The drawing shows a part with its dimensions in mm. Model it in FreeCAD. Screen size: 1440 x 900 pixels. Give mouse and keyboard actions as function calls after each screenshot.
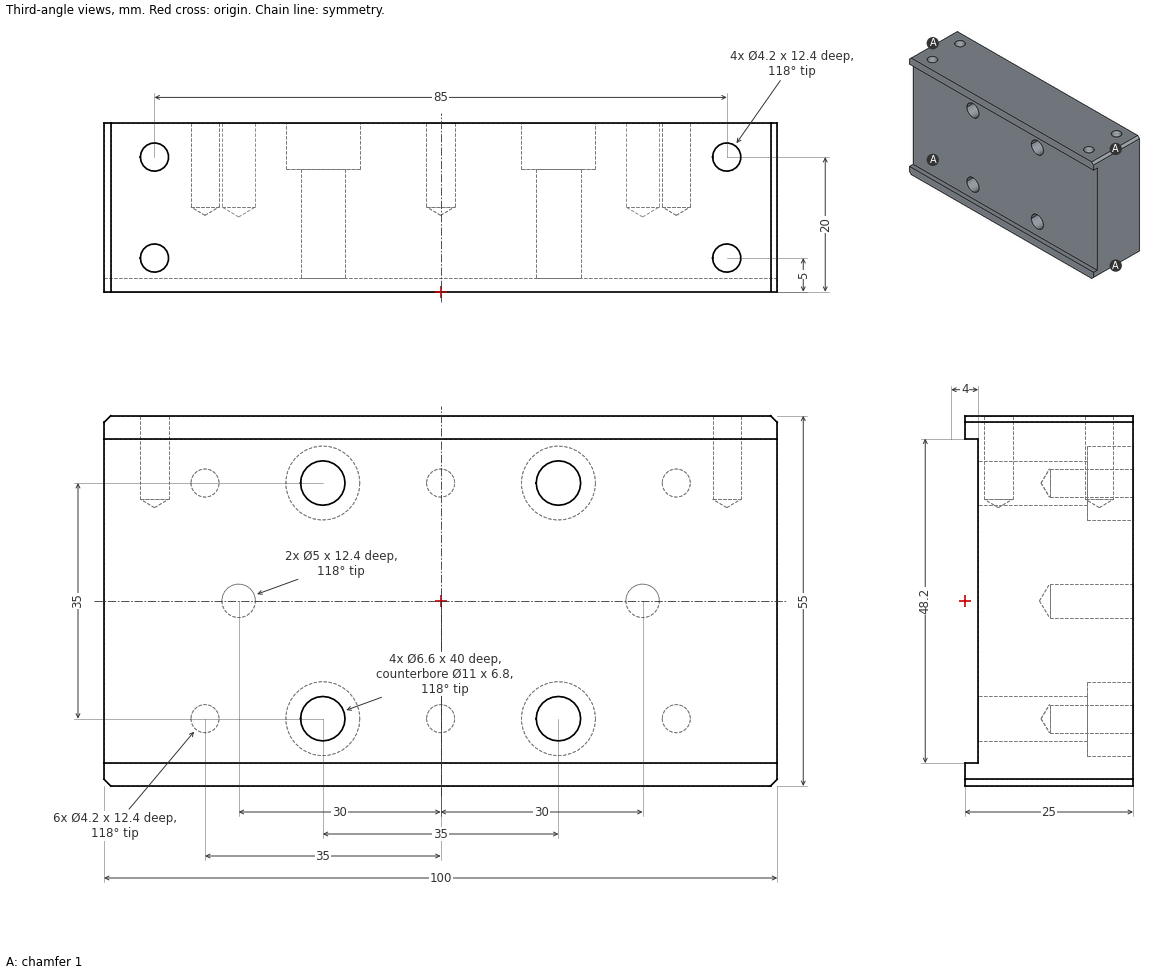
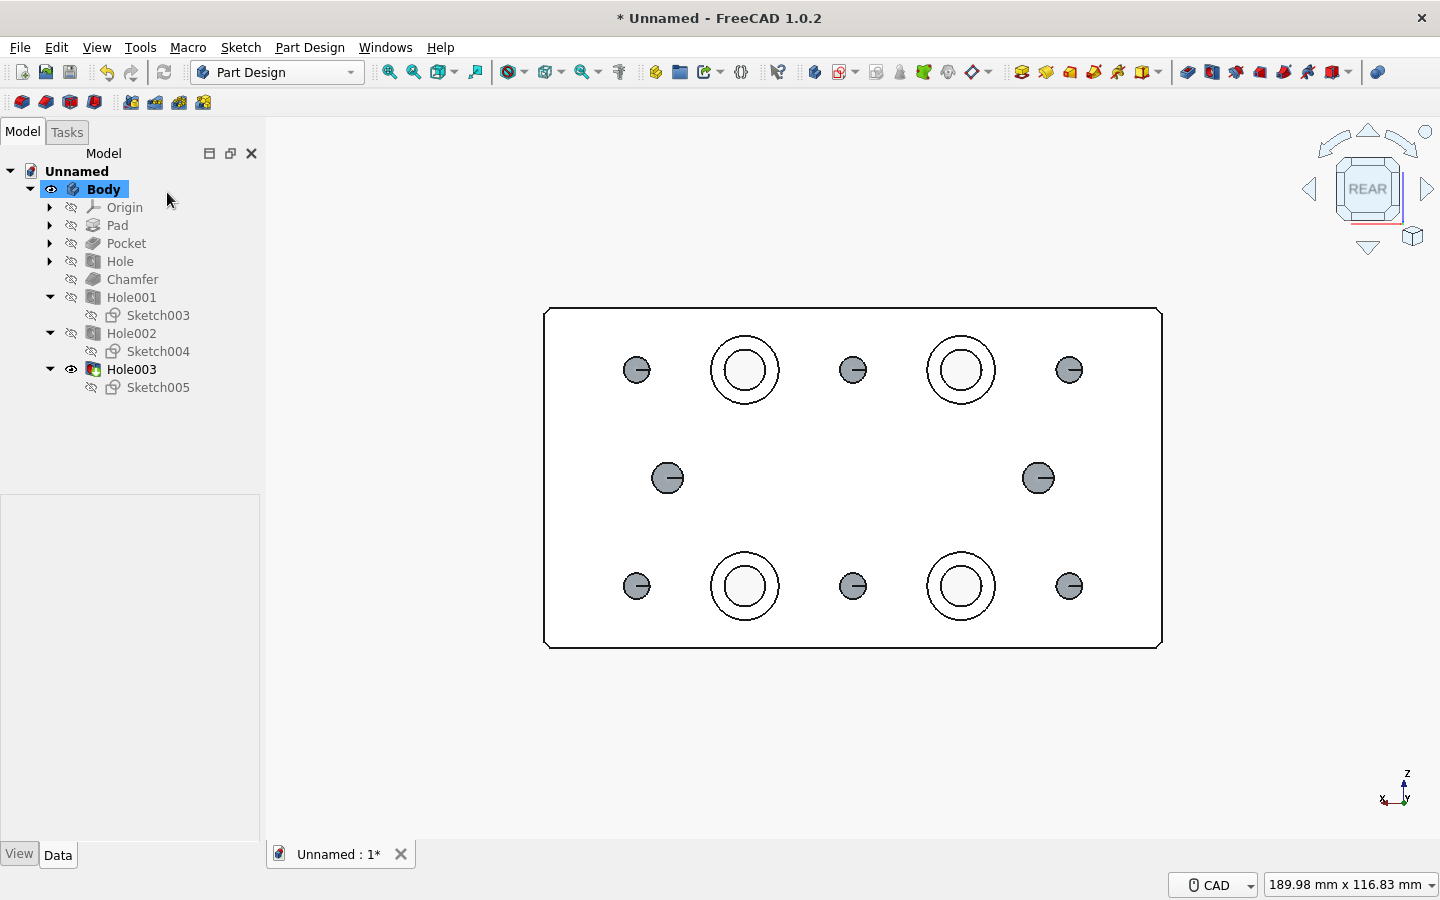
key(0)